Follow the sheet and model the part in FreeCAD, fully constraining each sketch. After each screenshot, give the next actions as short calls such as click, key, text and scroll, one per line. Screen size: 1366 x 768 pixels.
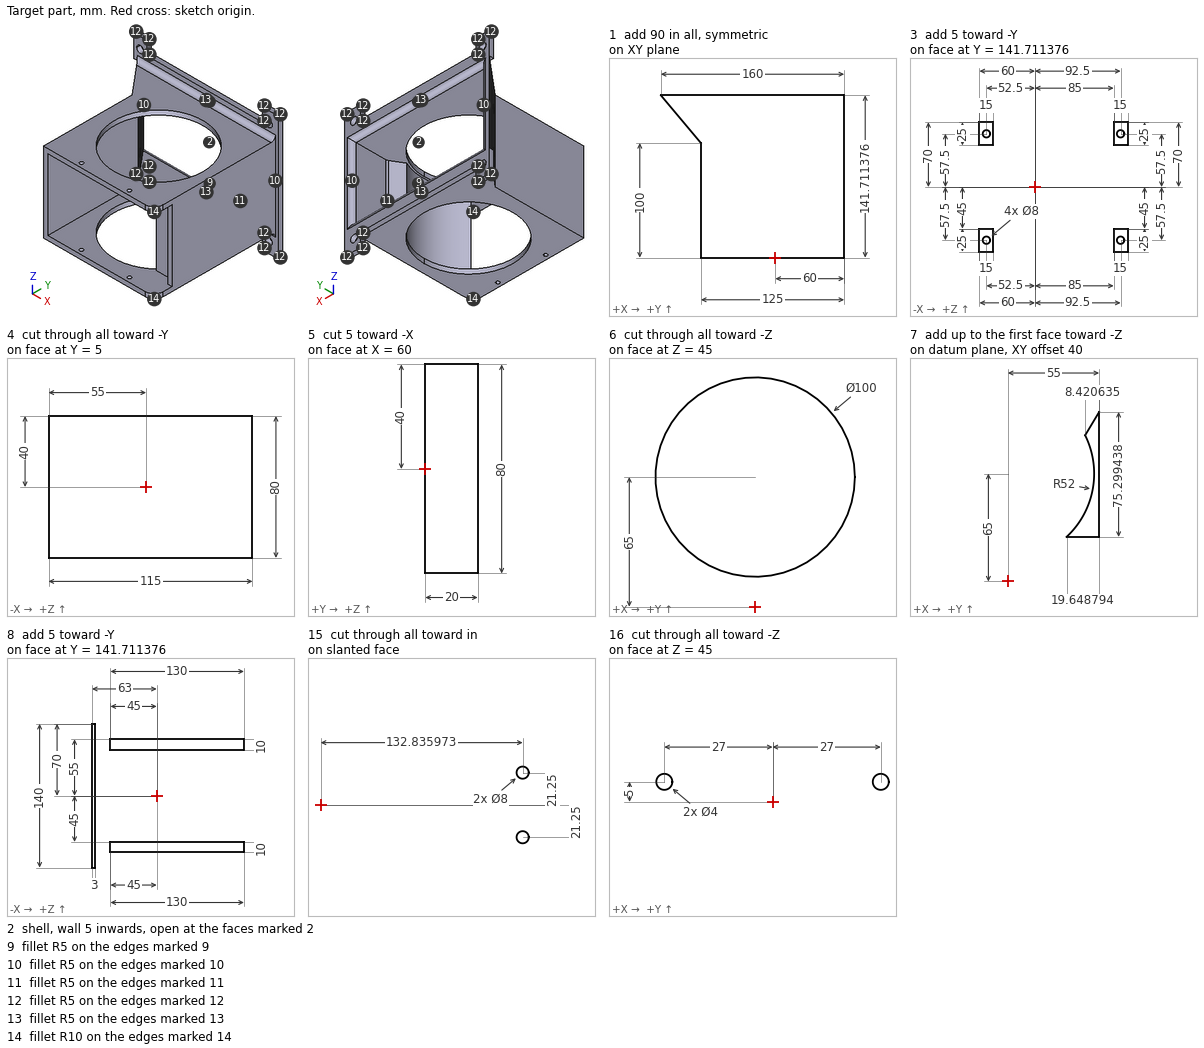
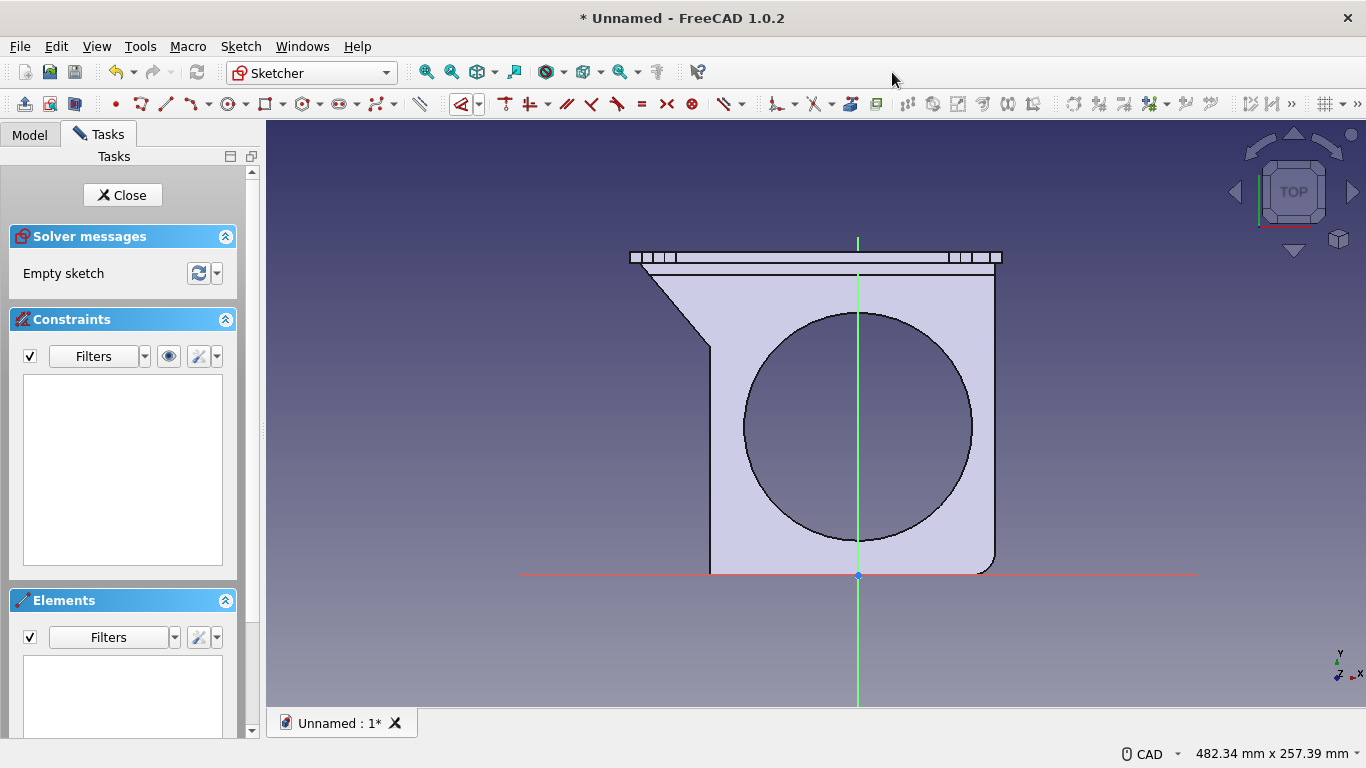
key(q)
key(s)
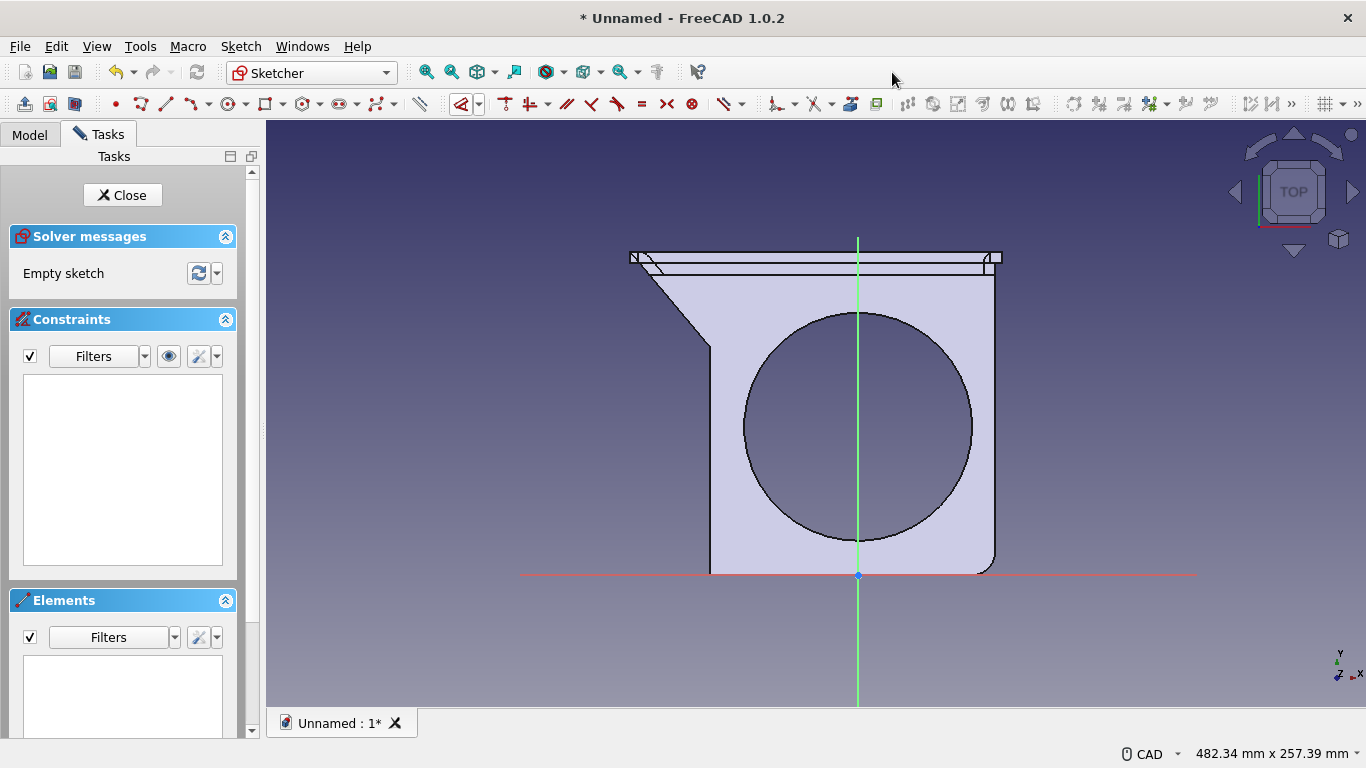
scroll(886, 606, up, 8)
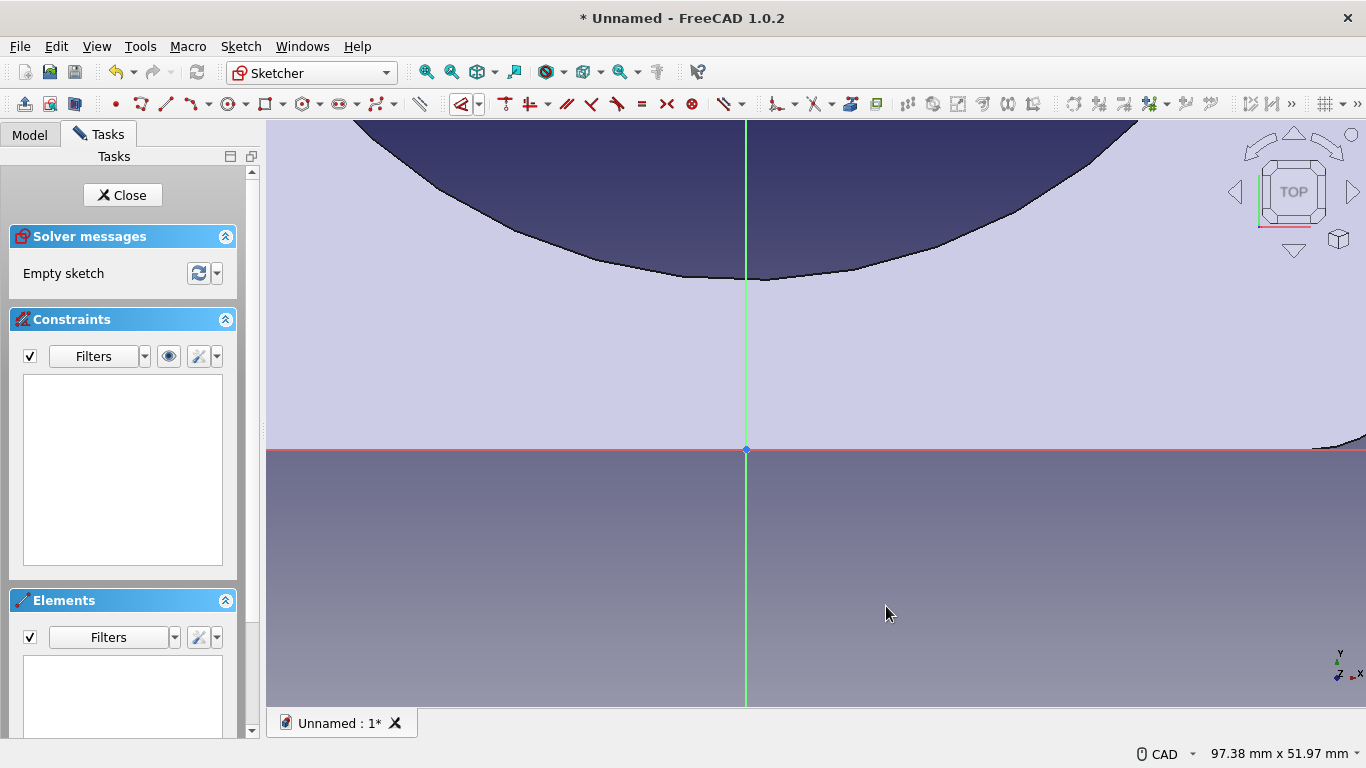
key(g)
key(c)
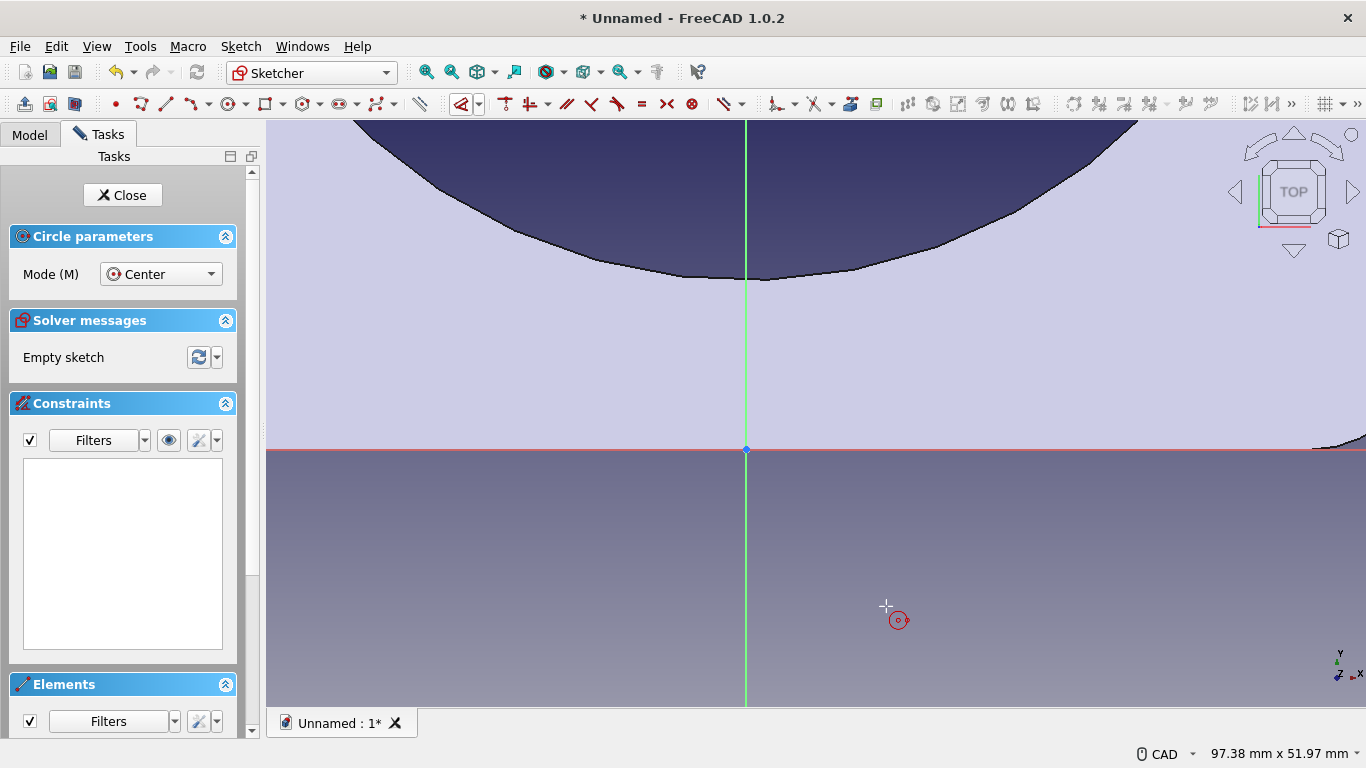
click(441, 393)
move(457, 377)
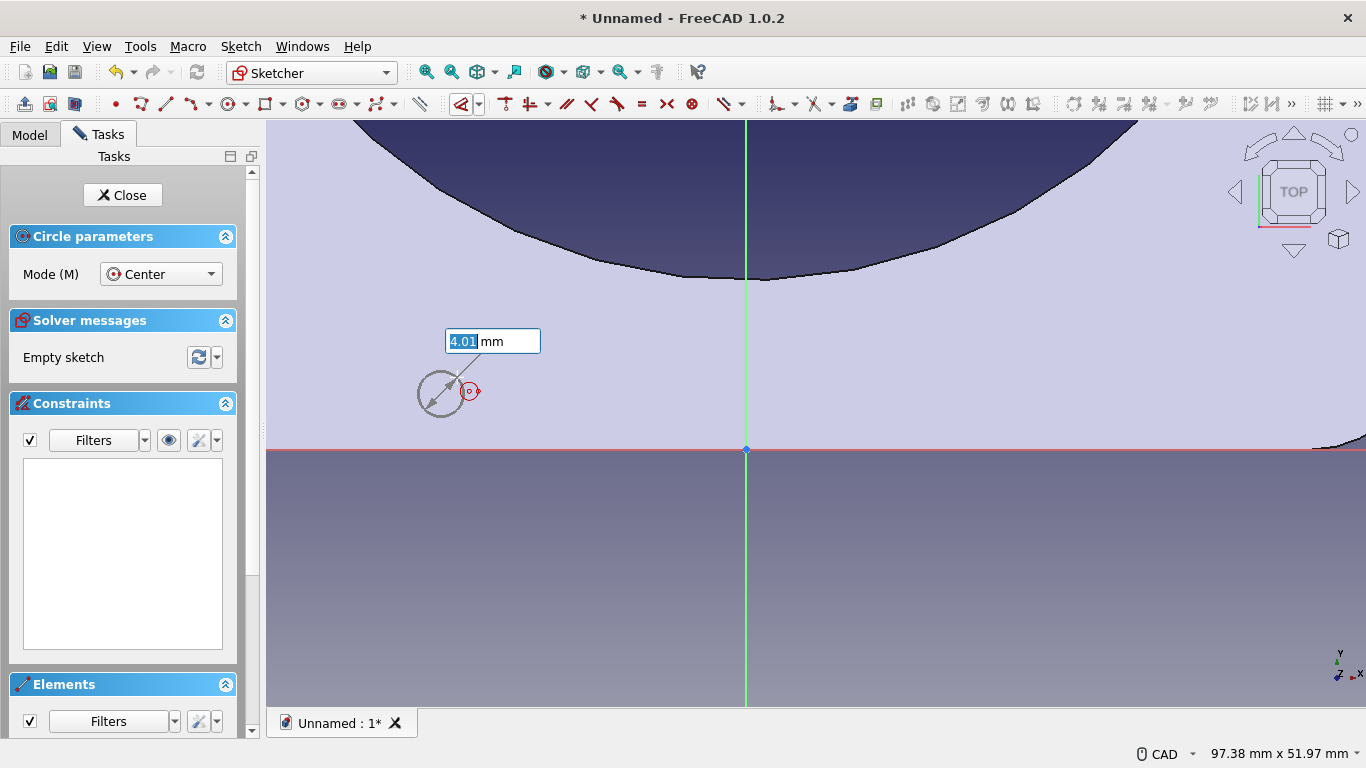
text(4)
key(Return)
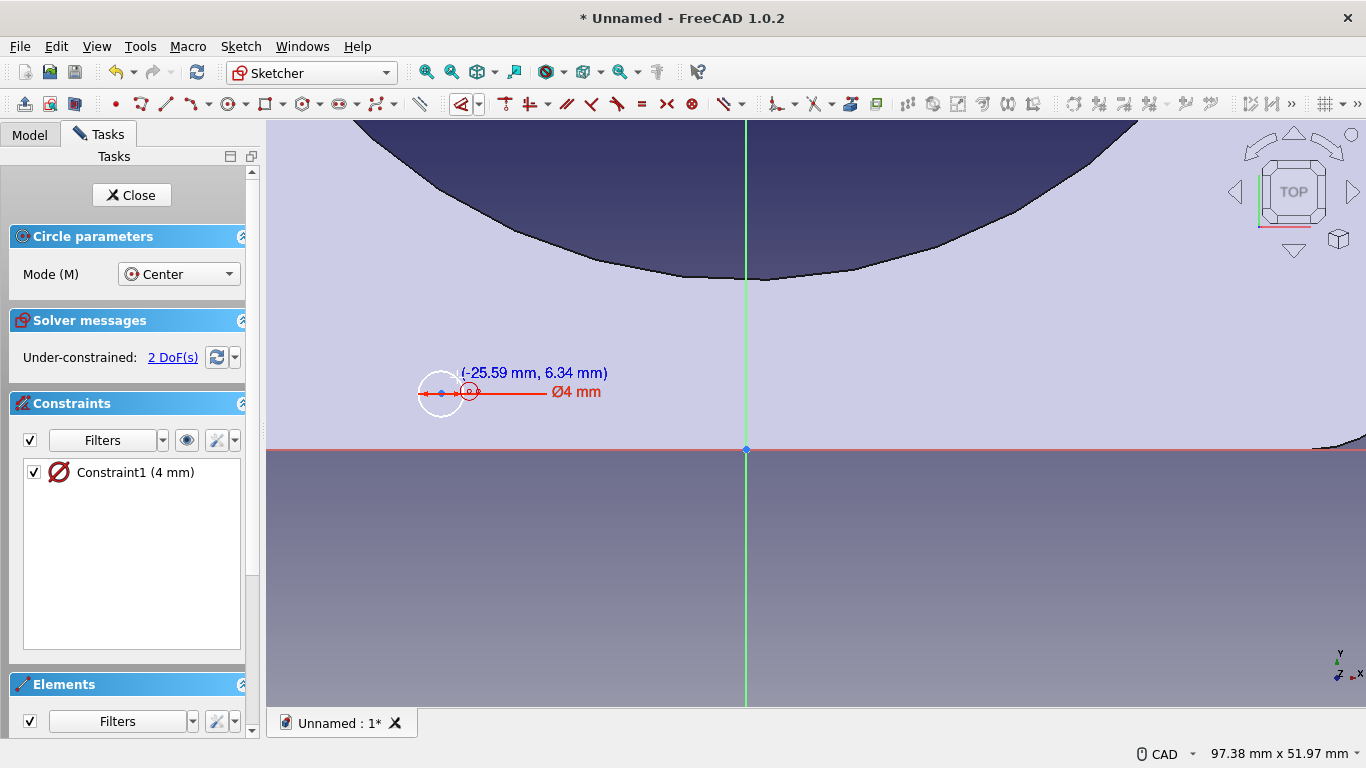
click(1051, 393)
move(1067, 377)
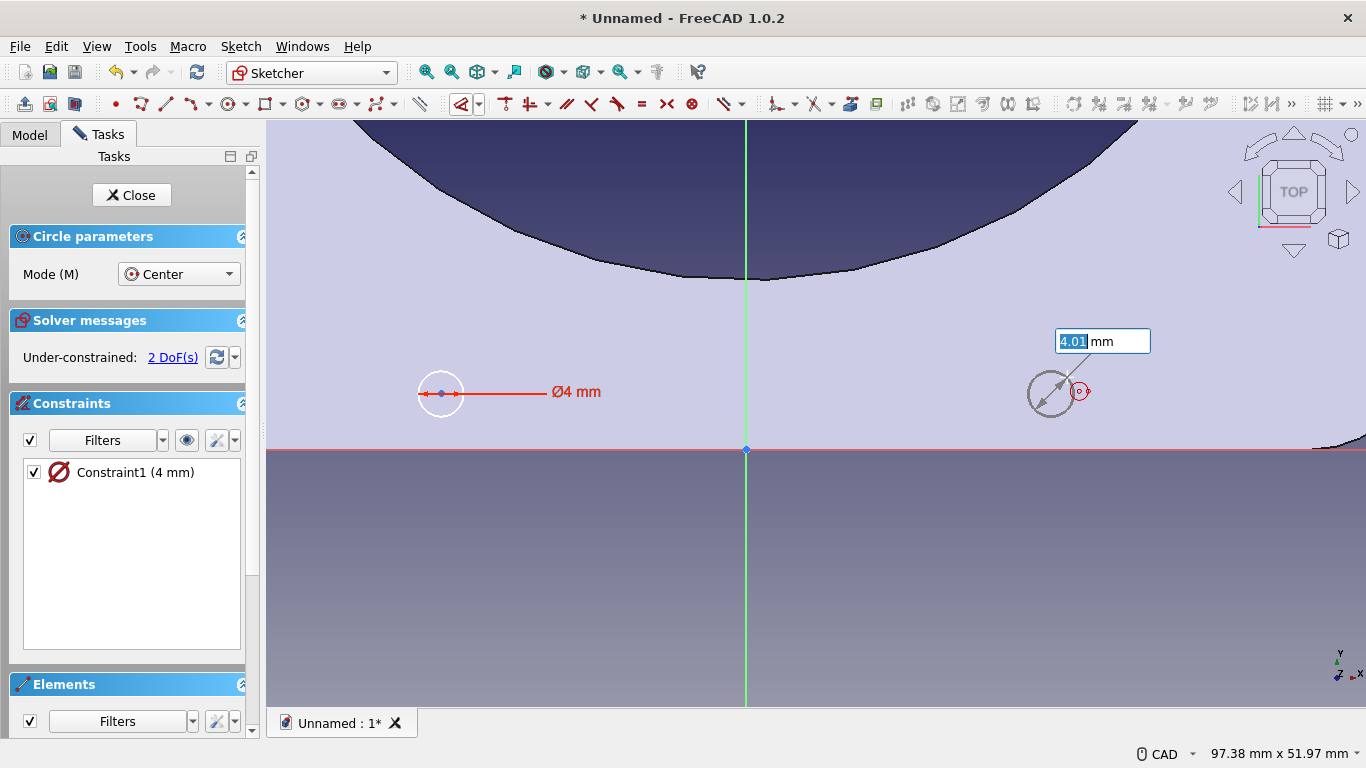
text(4)
key(Return)
key(Escape)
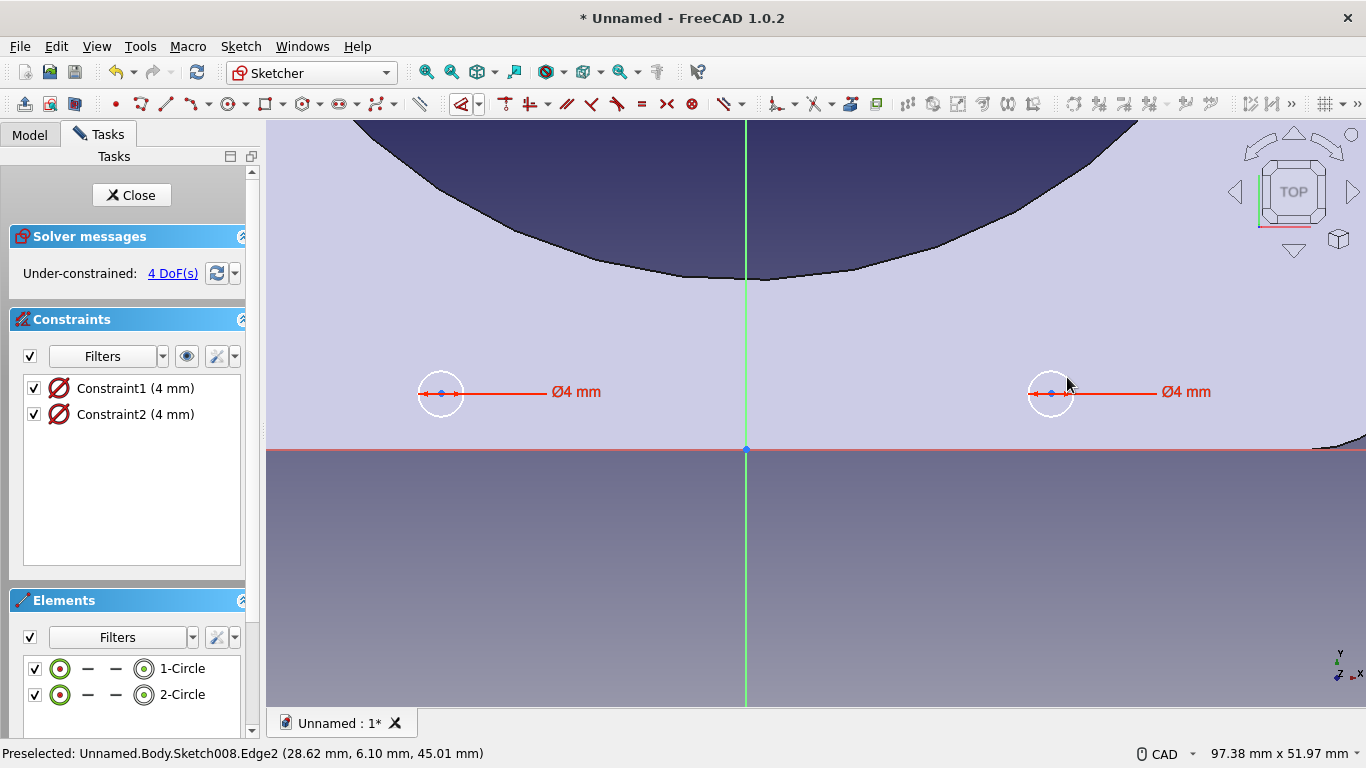
click(441, 394)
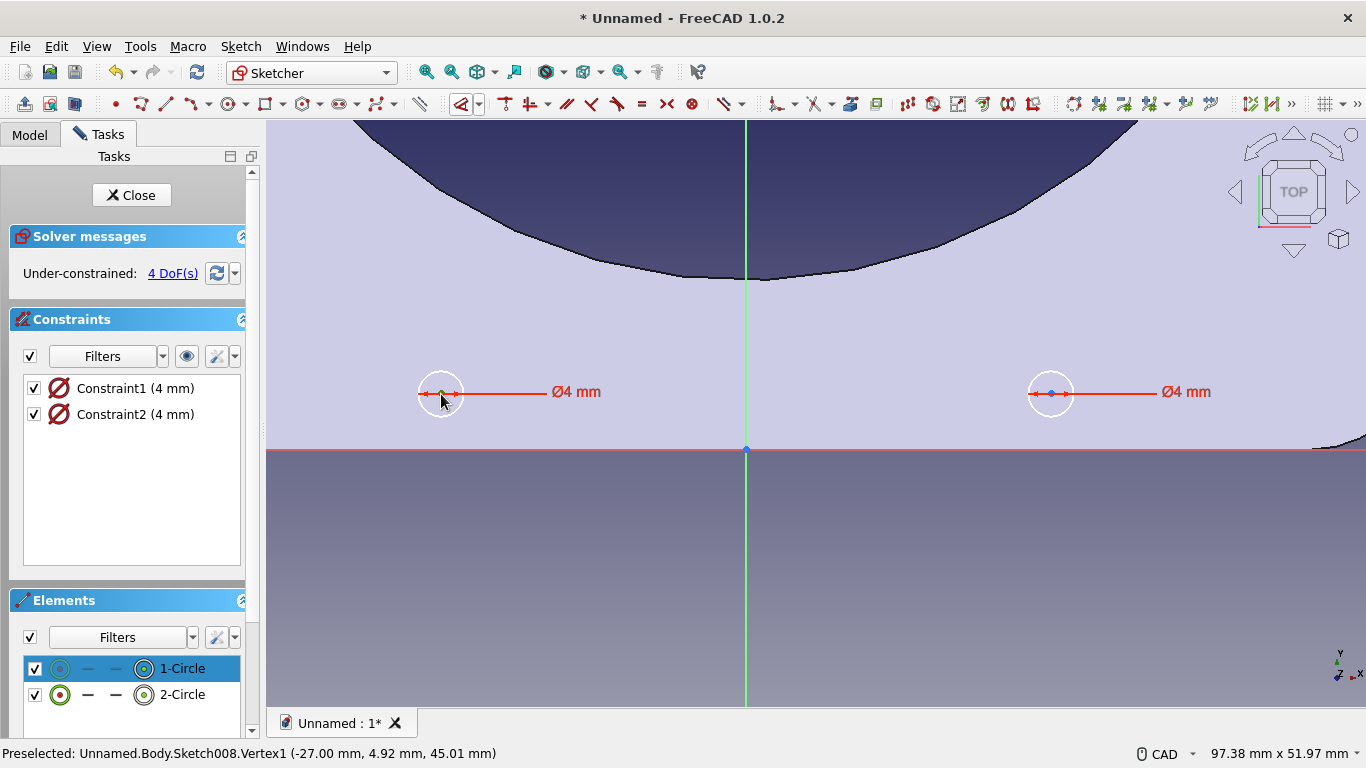
click(1051, 394)